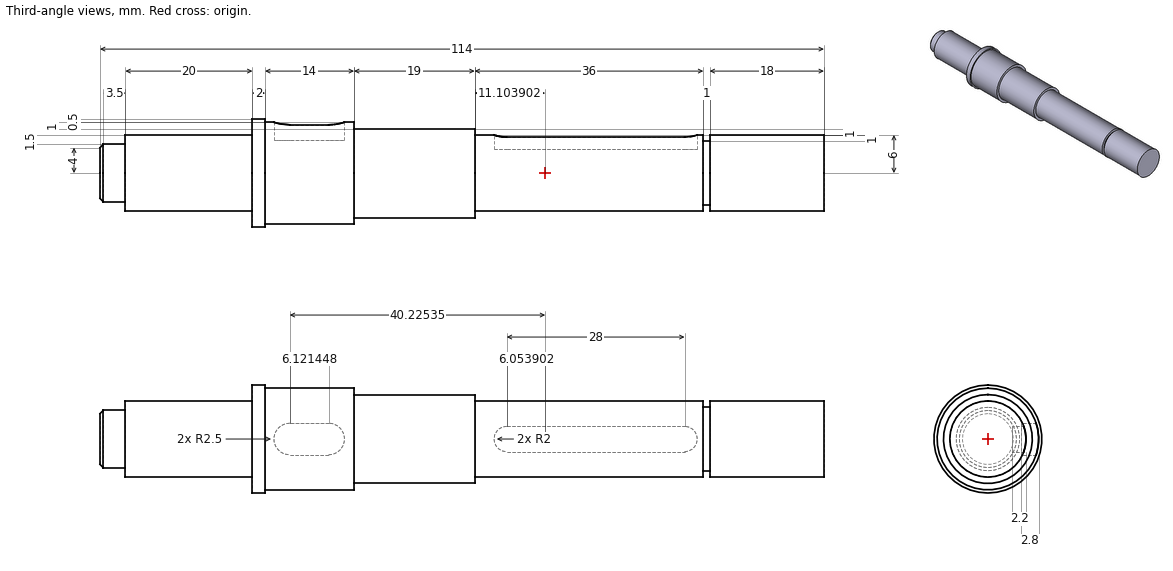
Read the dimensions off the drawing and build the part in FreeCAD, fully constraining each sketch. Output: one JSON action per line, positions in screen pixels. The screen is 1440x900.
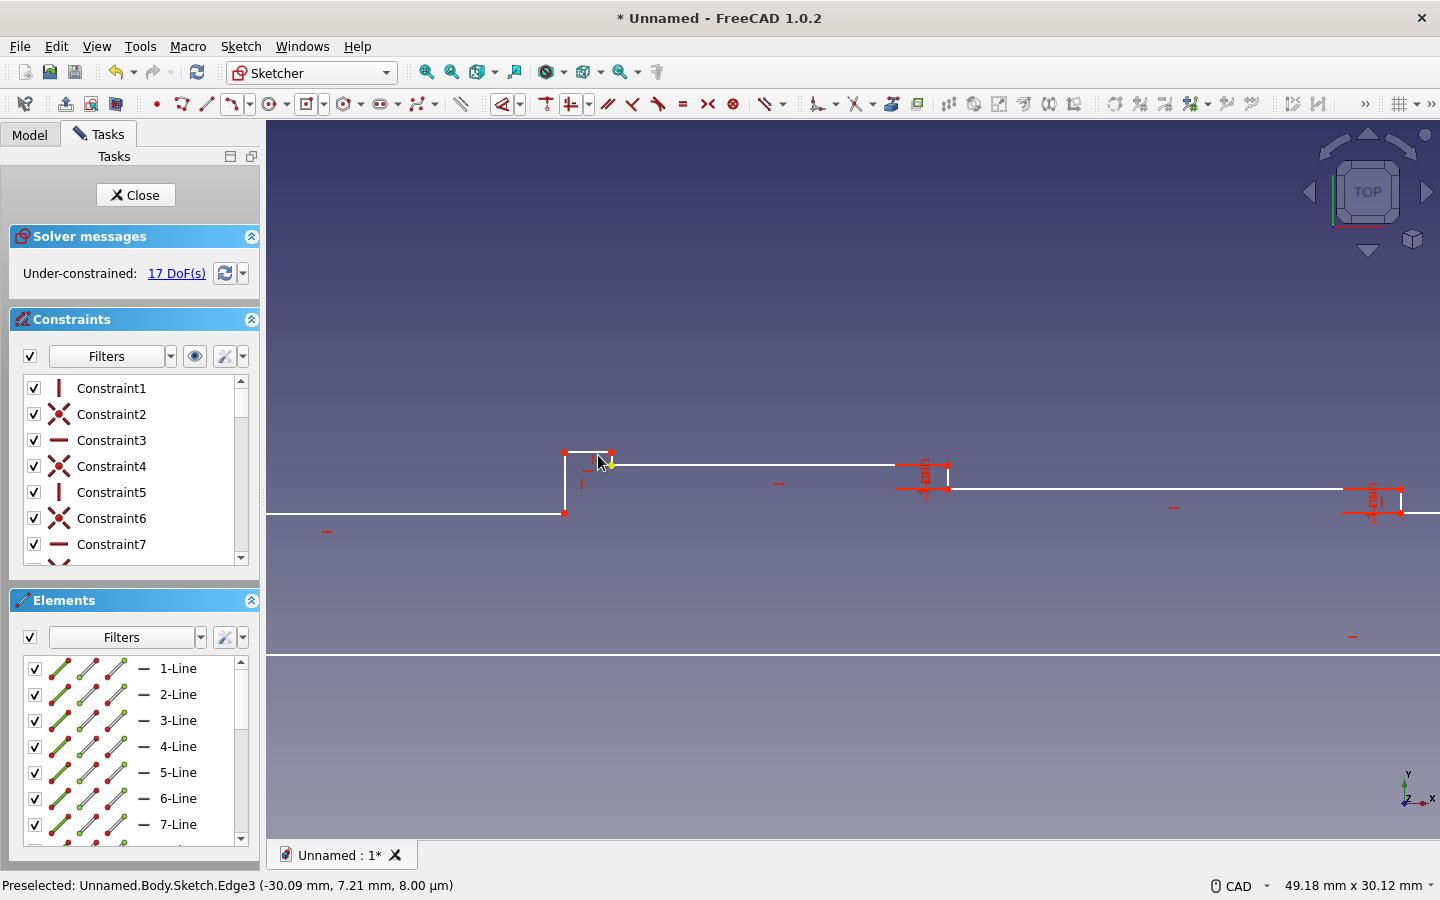
{"action": "left_click", "coordinate": [579, 452]}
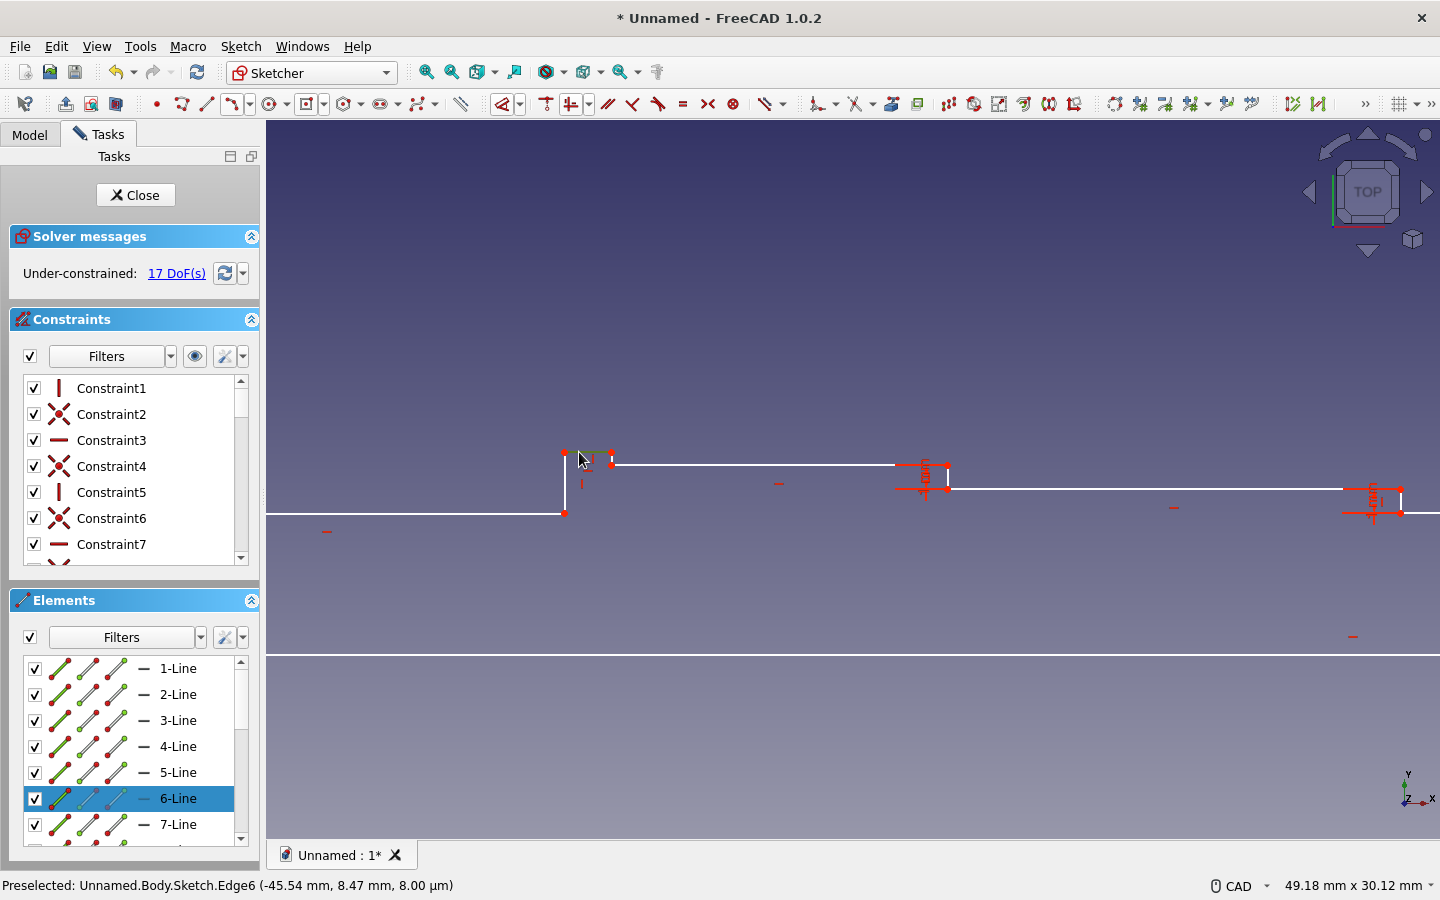
{"action": "key", "text": "l"}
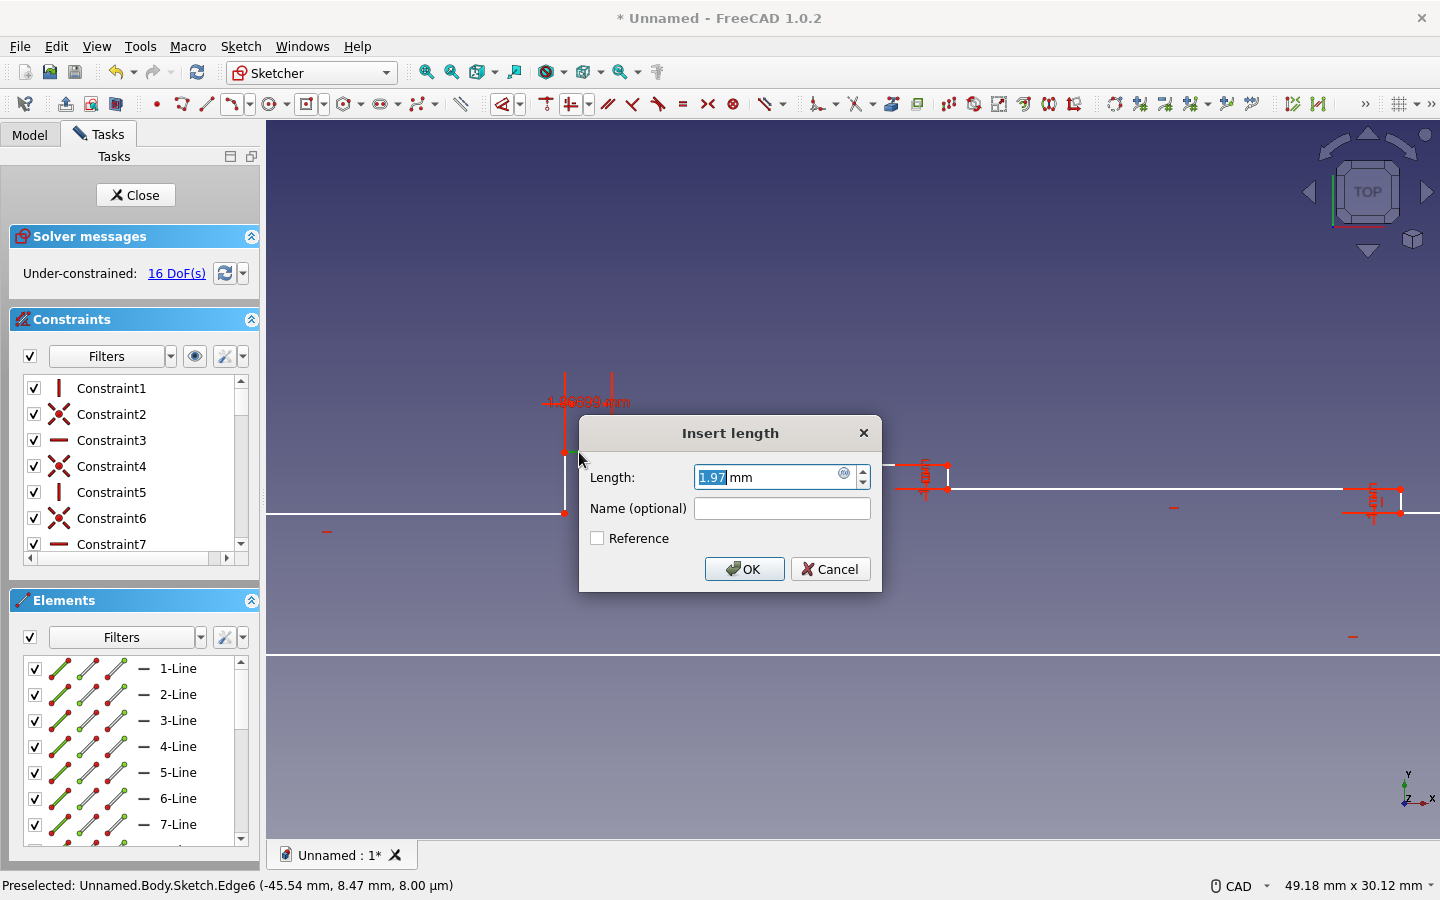
{"action": "type", "text": "2"}
{"action": "key", "text": "Return"}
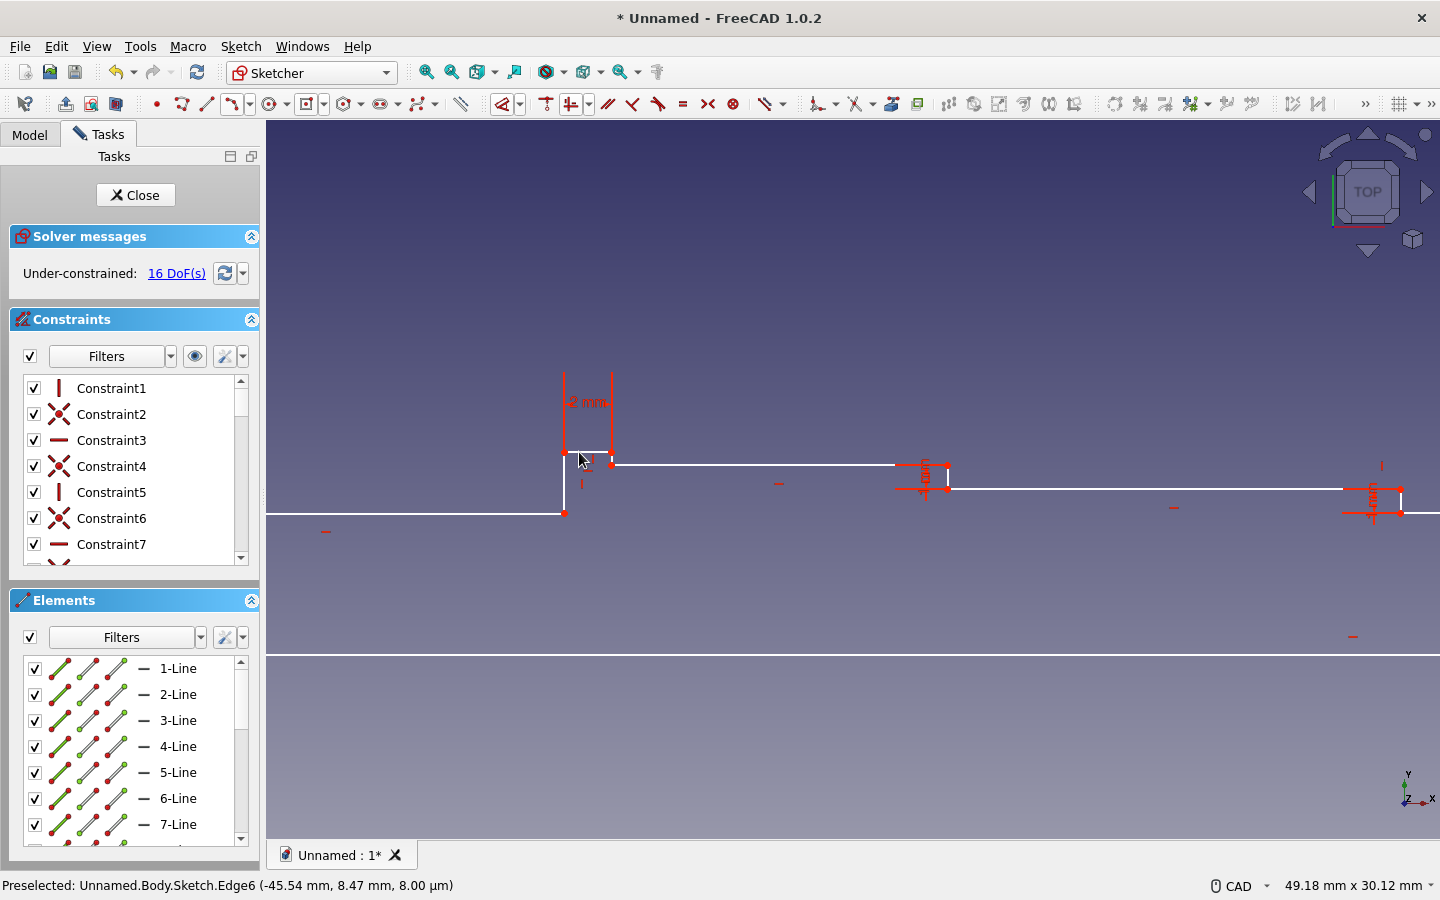
{"action": "scroll", "coordinate": [598, 455], "scroll_direction": "down", "scroll_amount": 7}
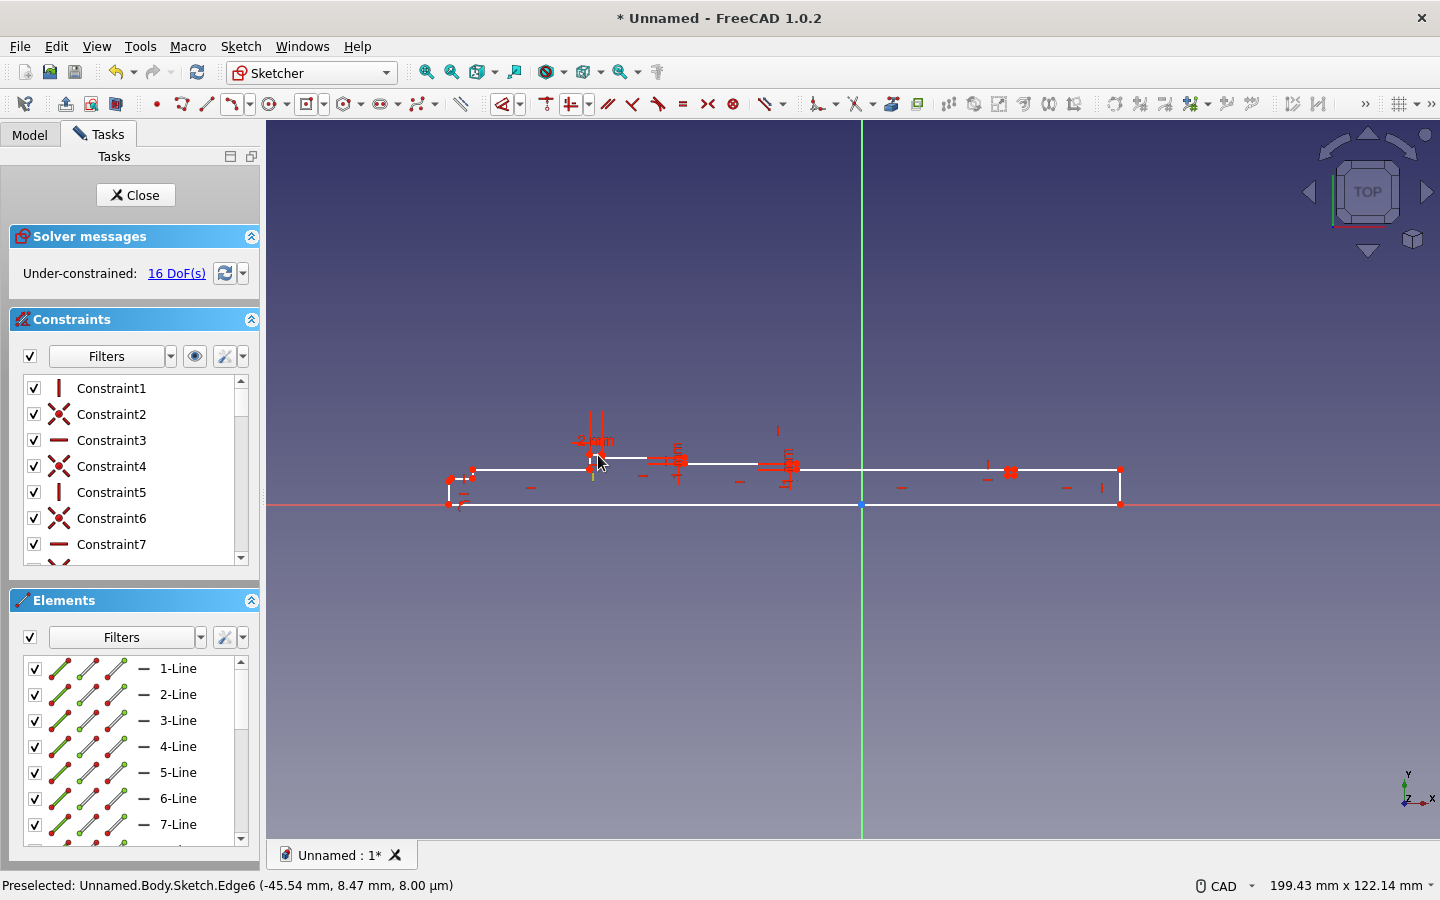
{"action": "scroll", "coordinate": [449, 488], "scroll_direction": "up", "scroll_amount": 4}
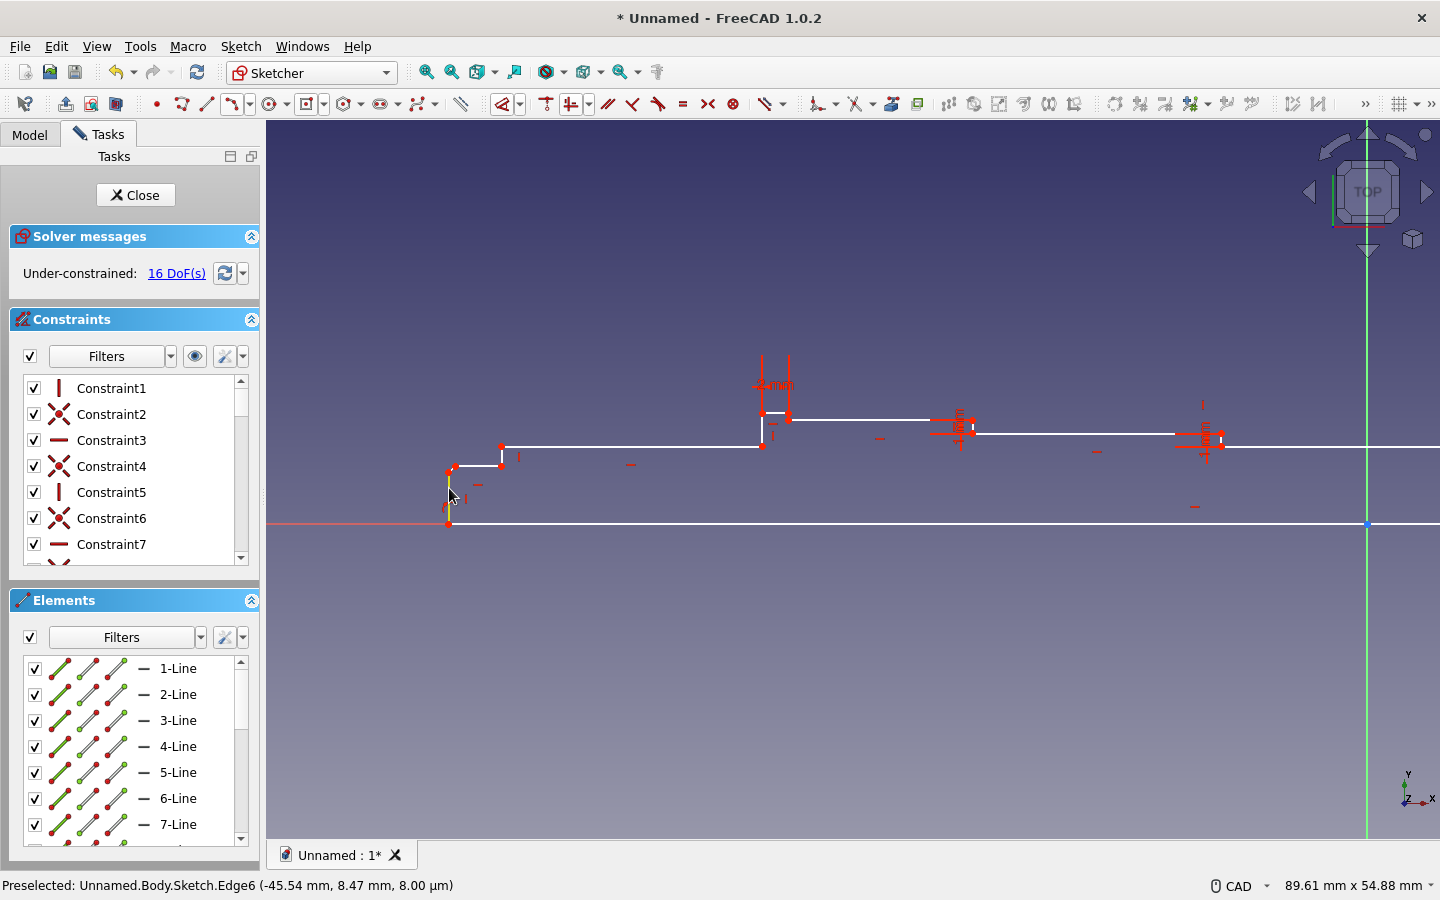
{"action": "left_click", "coordinate": [449, 488]}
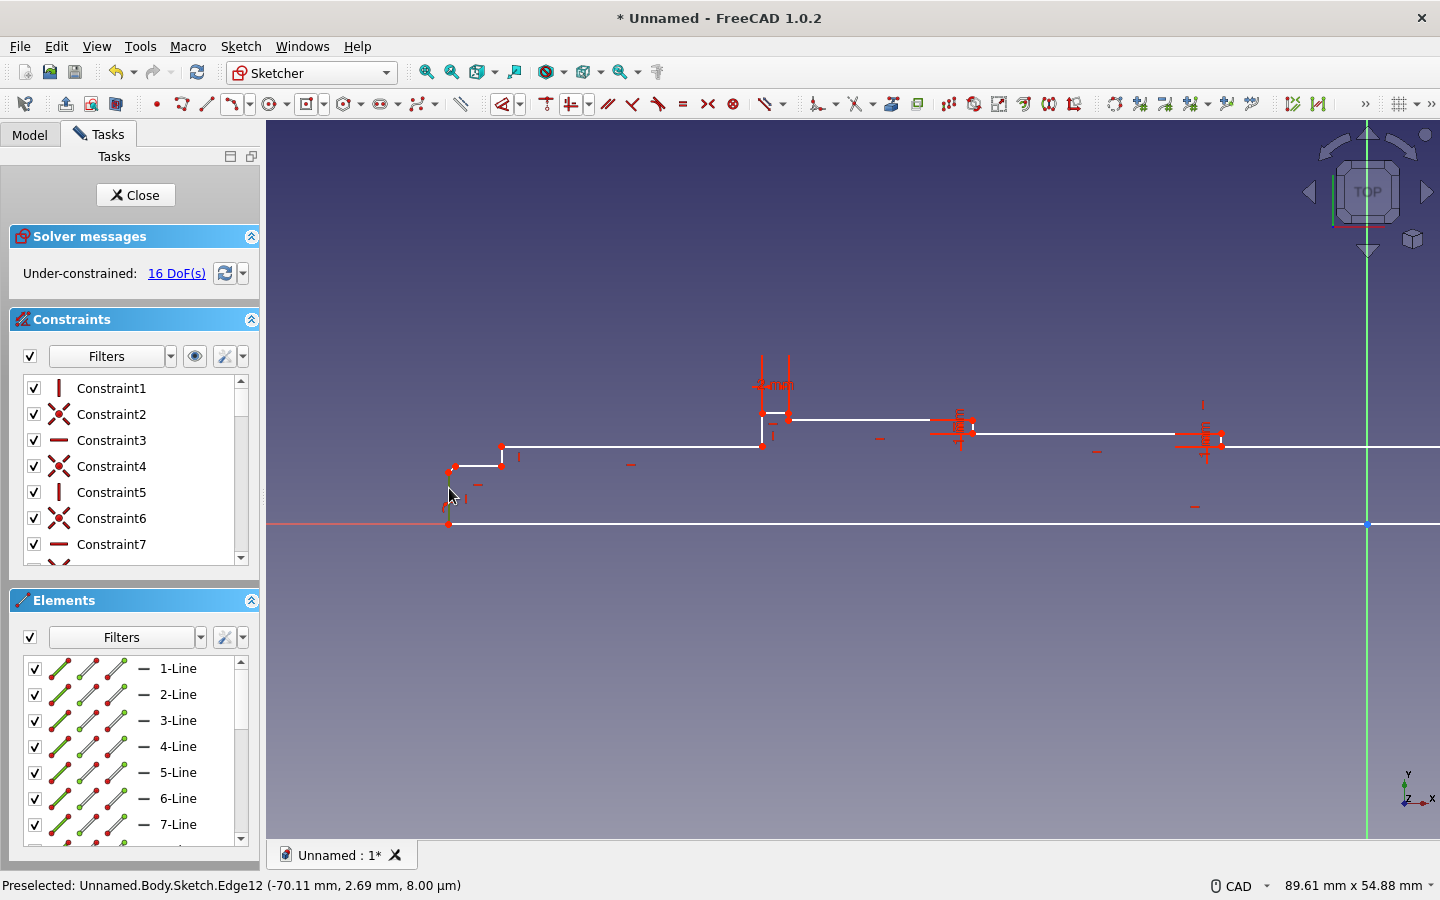
{"action": "left_click", "coordinate": [520, 104]}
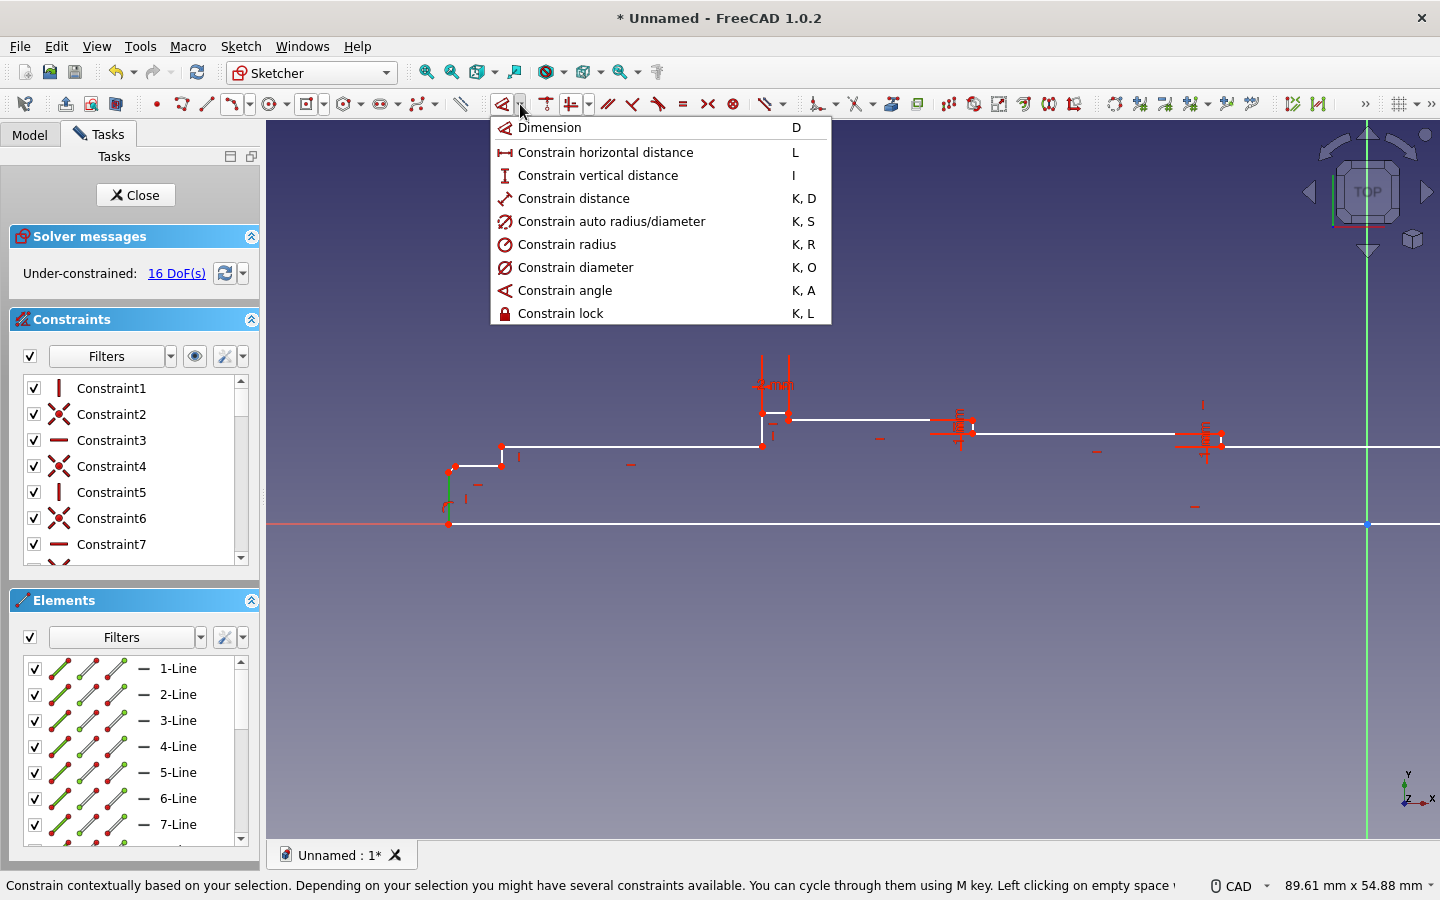
{"action": "left_click", "coordinate": [661, 176]}